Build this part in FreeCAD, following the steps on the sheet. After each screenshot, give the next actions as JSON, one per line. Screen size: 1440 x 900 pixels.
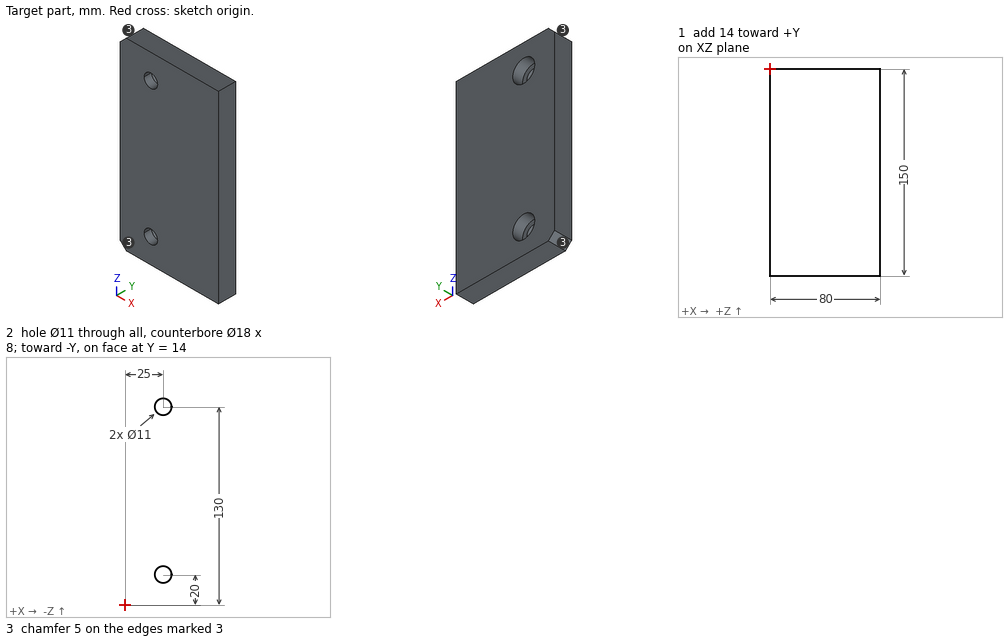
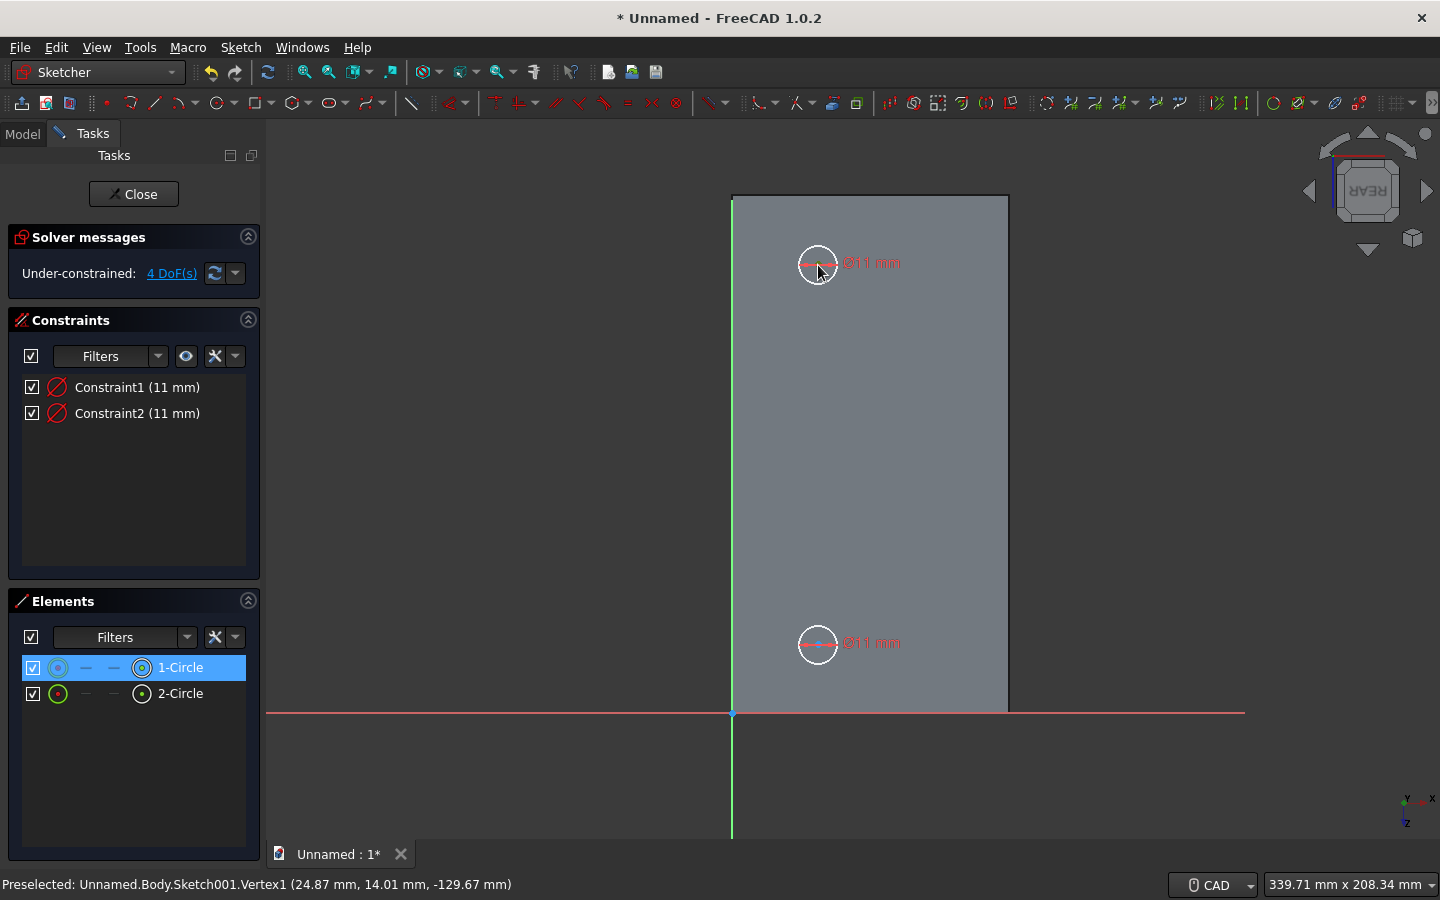
{"action": "left_click", "coordinate": [818, 645]}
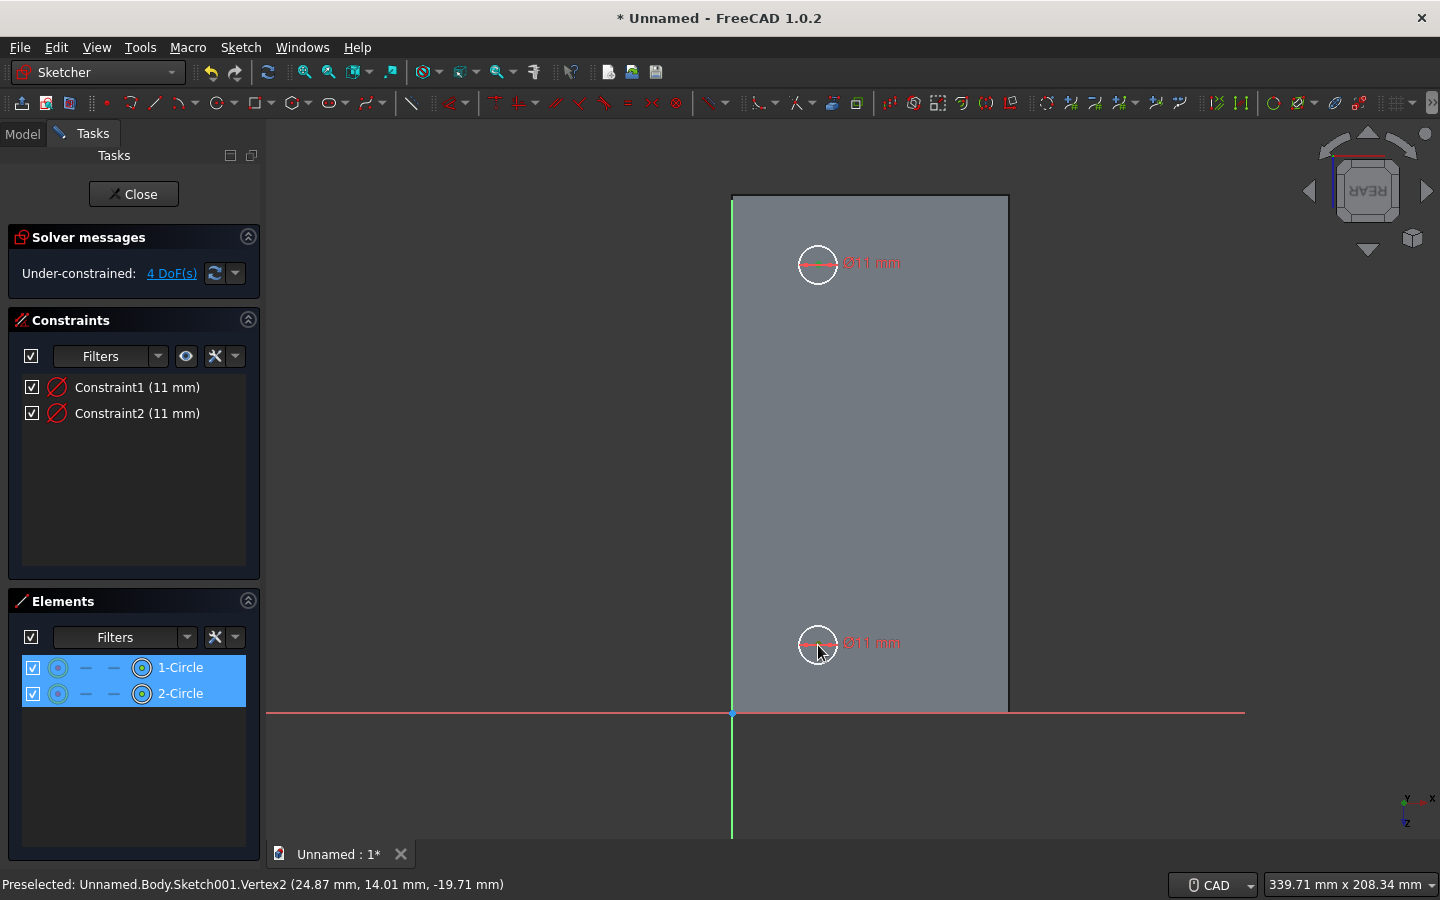
{"action": "key", "text": "v"}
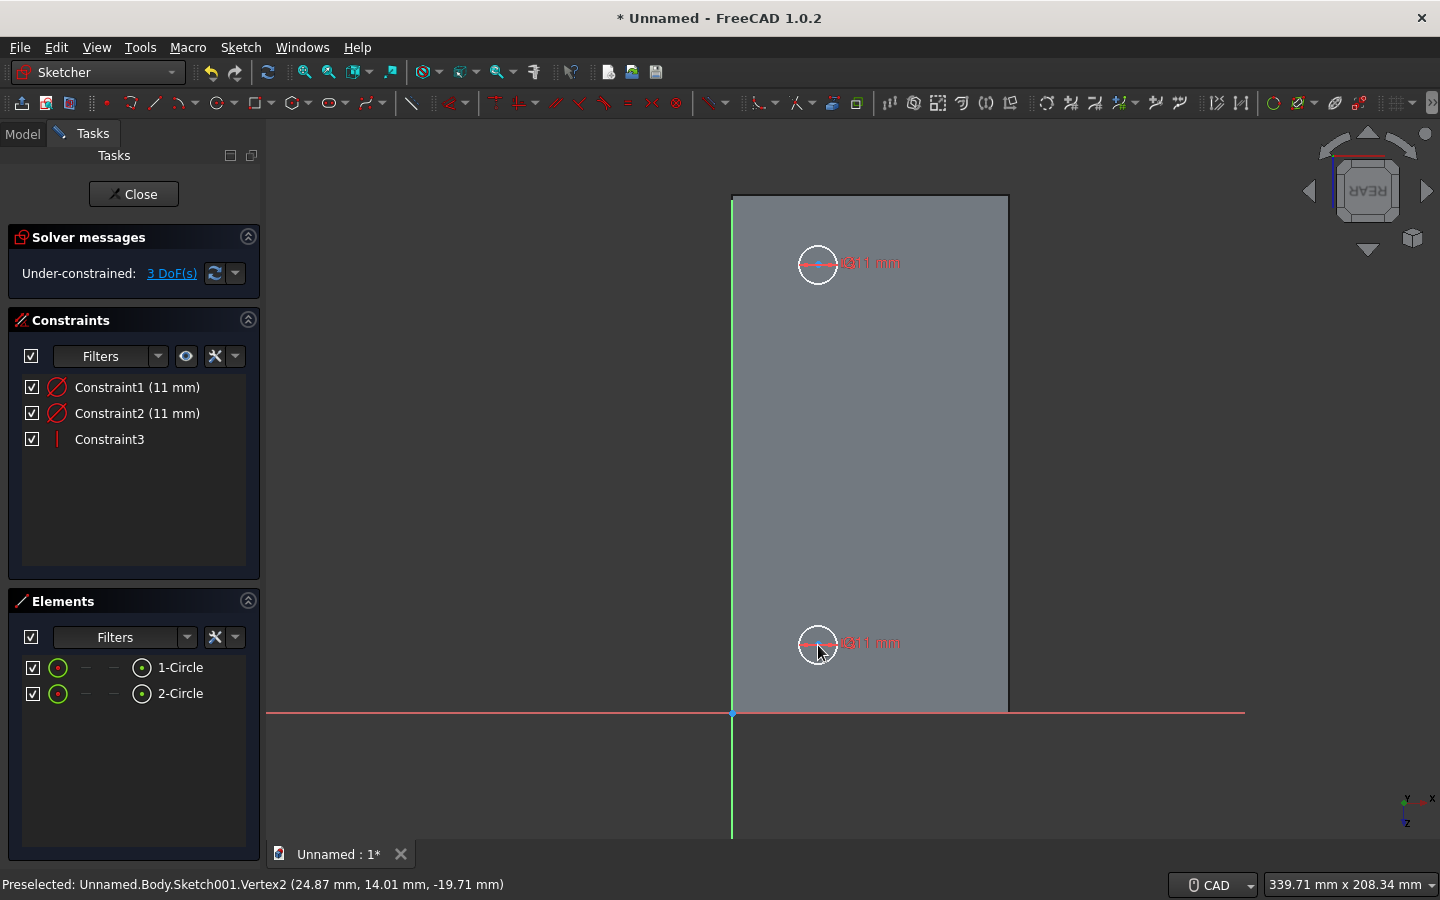
{"action": "key", "text": "d"}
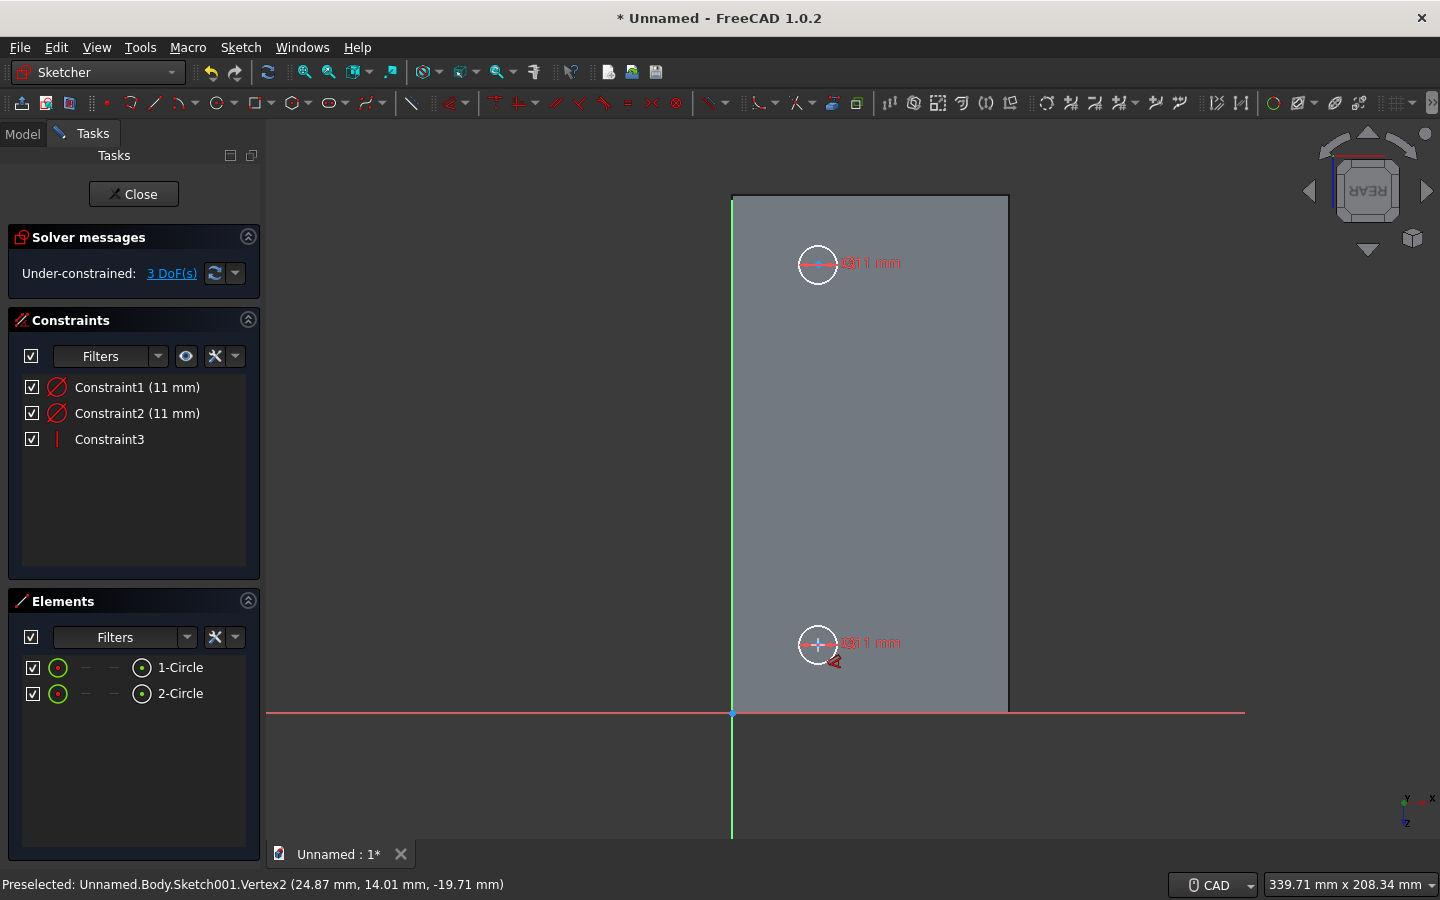
{"action": "left_click", "coordinate": [818, 265]}
{"action": "left_click", "coordinate": [775, 747]}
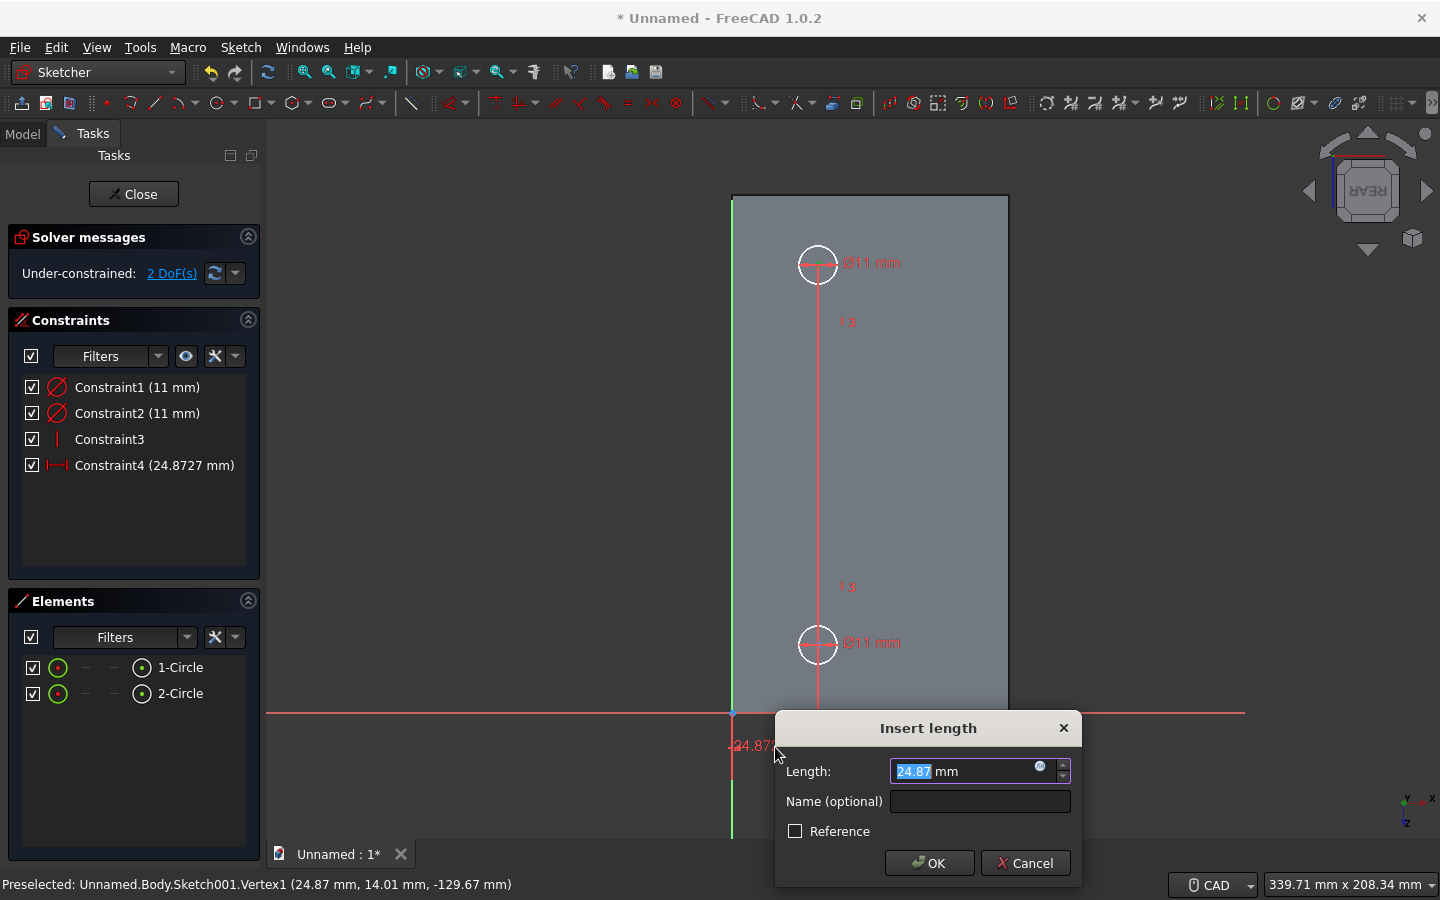
{"action": "type", "text": "25"}
{"action": "key", "text": "Return"}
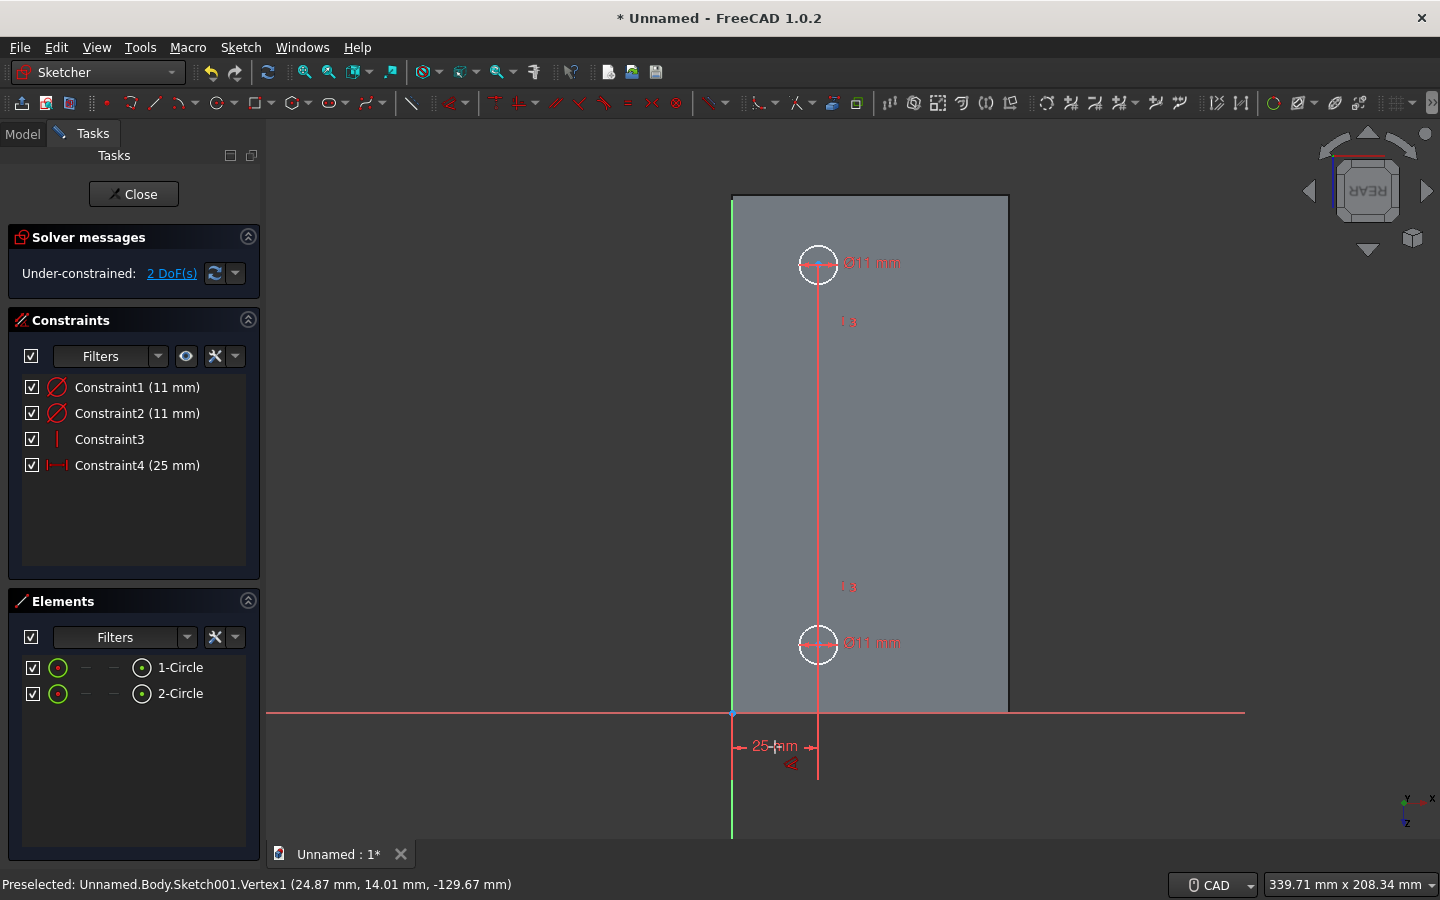
{"action": "left_click", "coordinate": [818, 645]}
{"action": "left_click", "coordinate": [698, 679]}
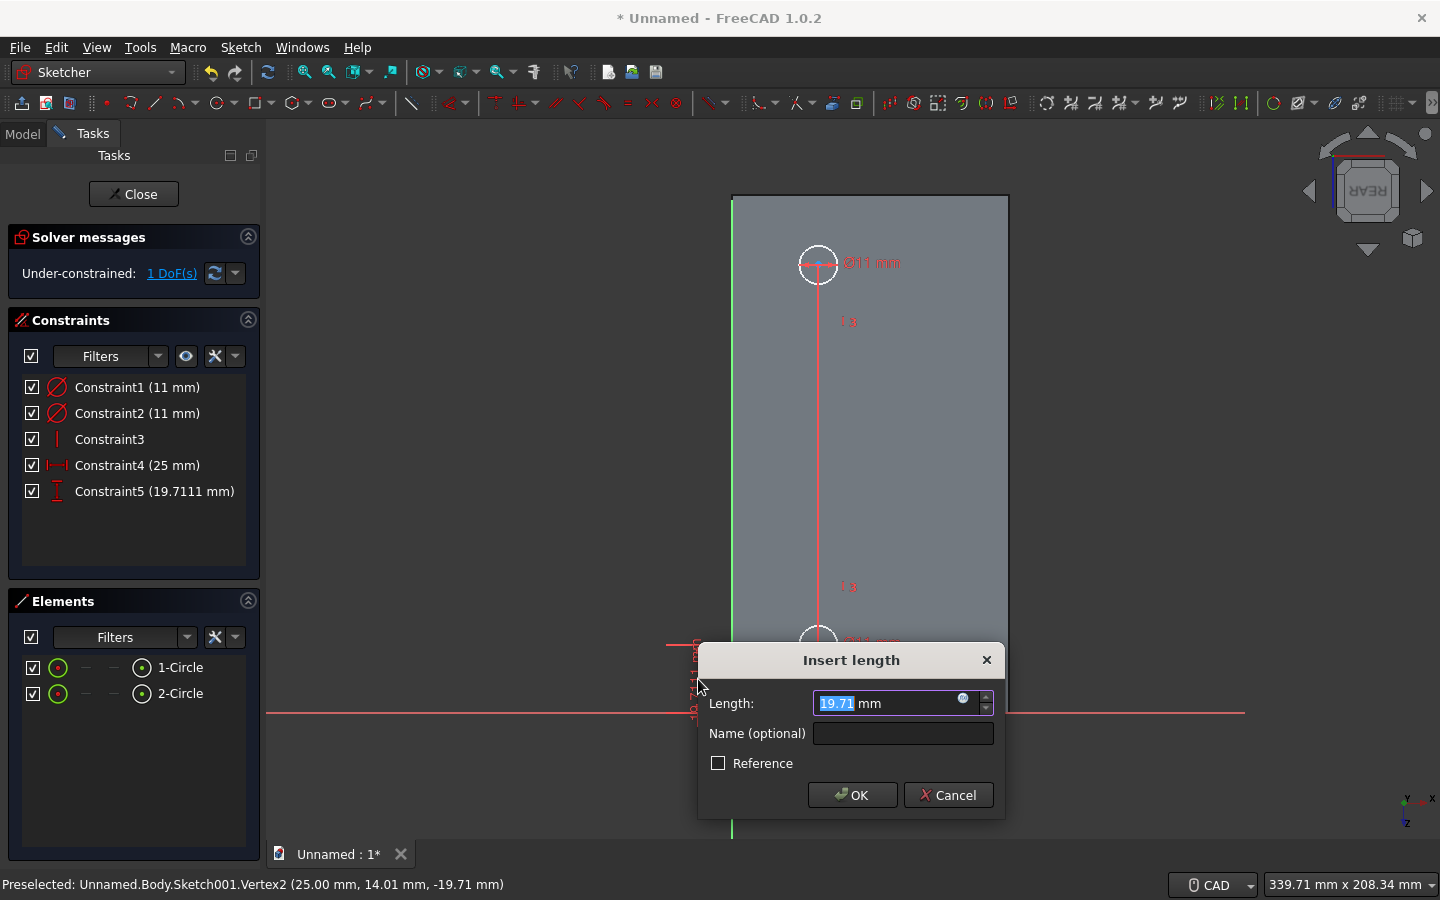
{"action": "type", "text": "20"}
{"action": "key", "text": "Return"}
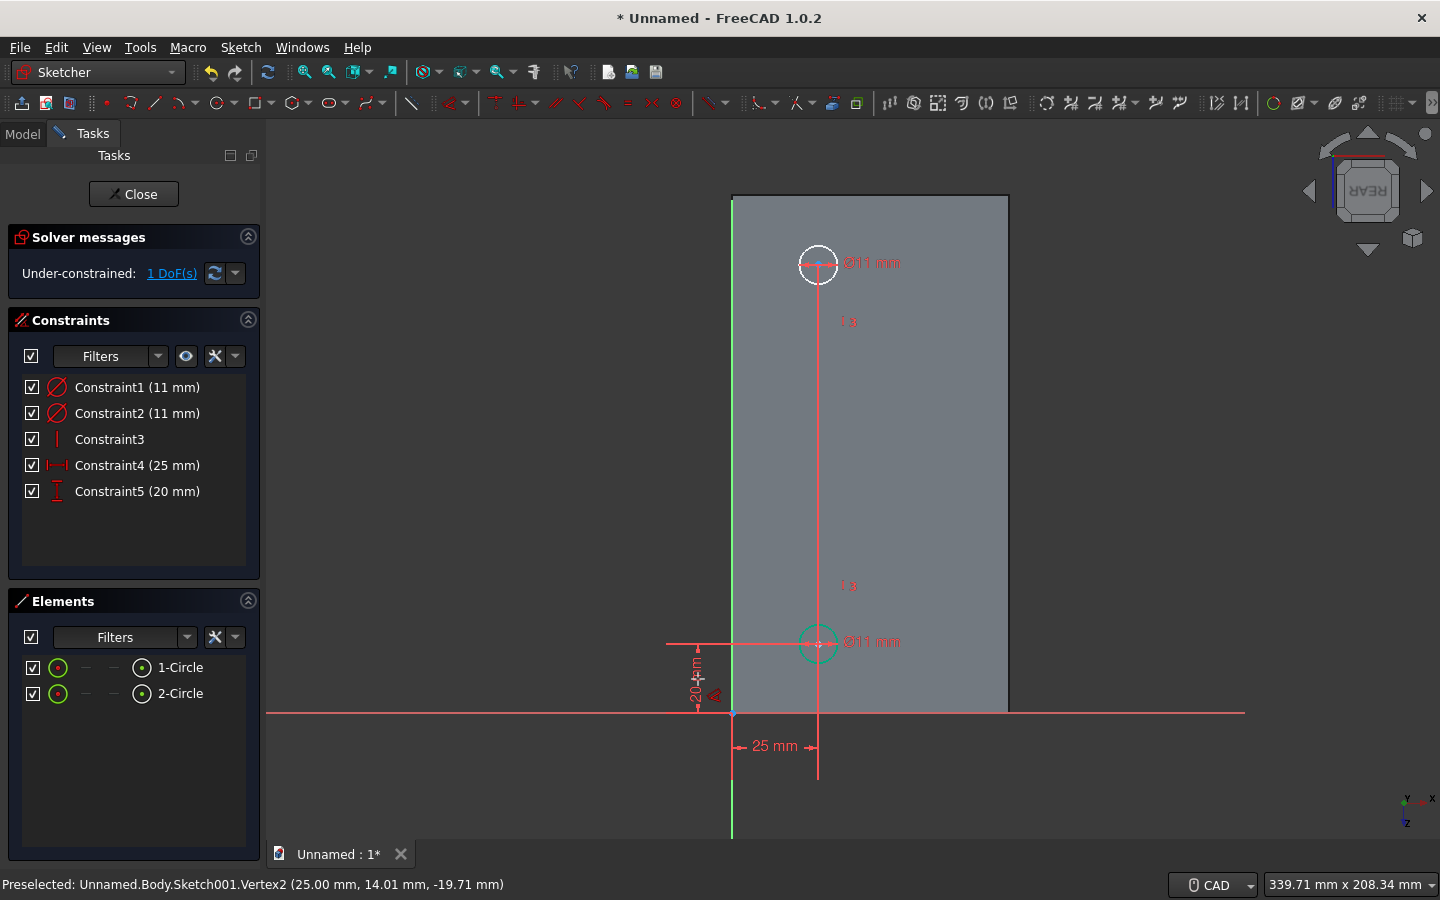
{"action": "left_click", "coordinate": [818, 265]}
{"action": "left_click", "coordinate": [698, 489]}